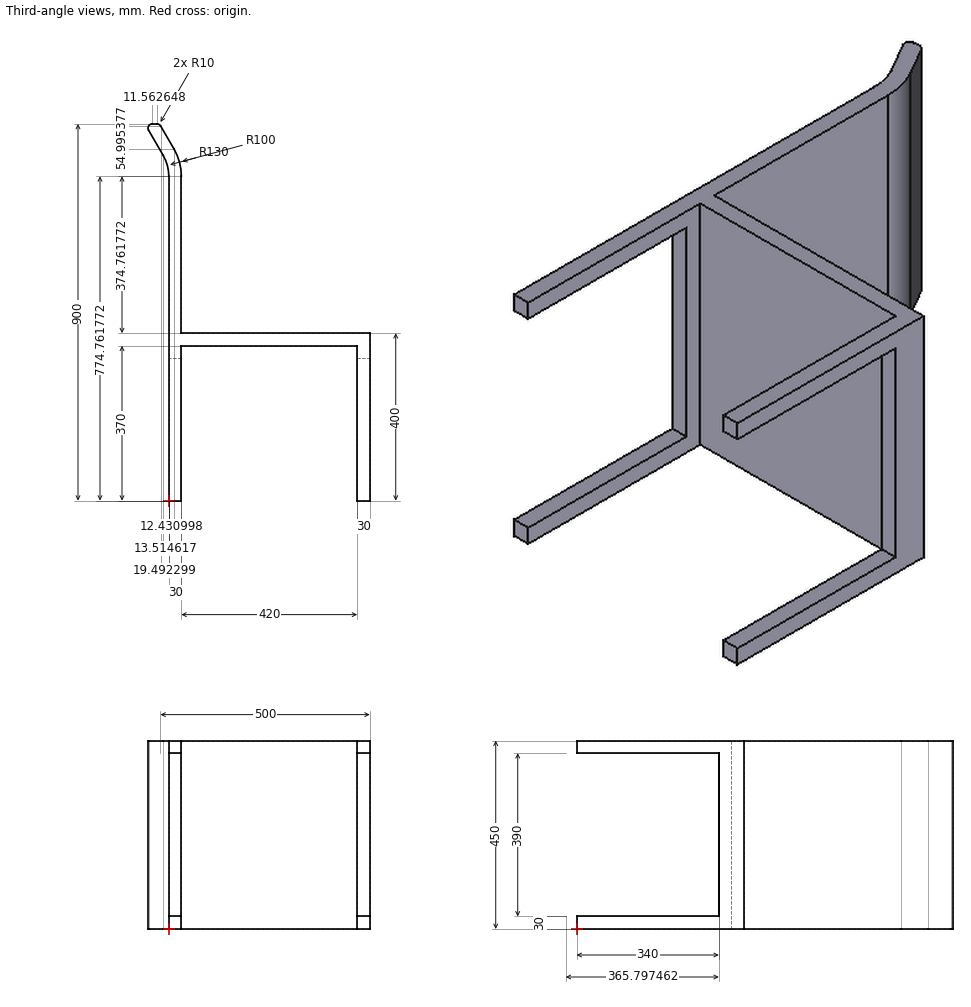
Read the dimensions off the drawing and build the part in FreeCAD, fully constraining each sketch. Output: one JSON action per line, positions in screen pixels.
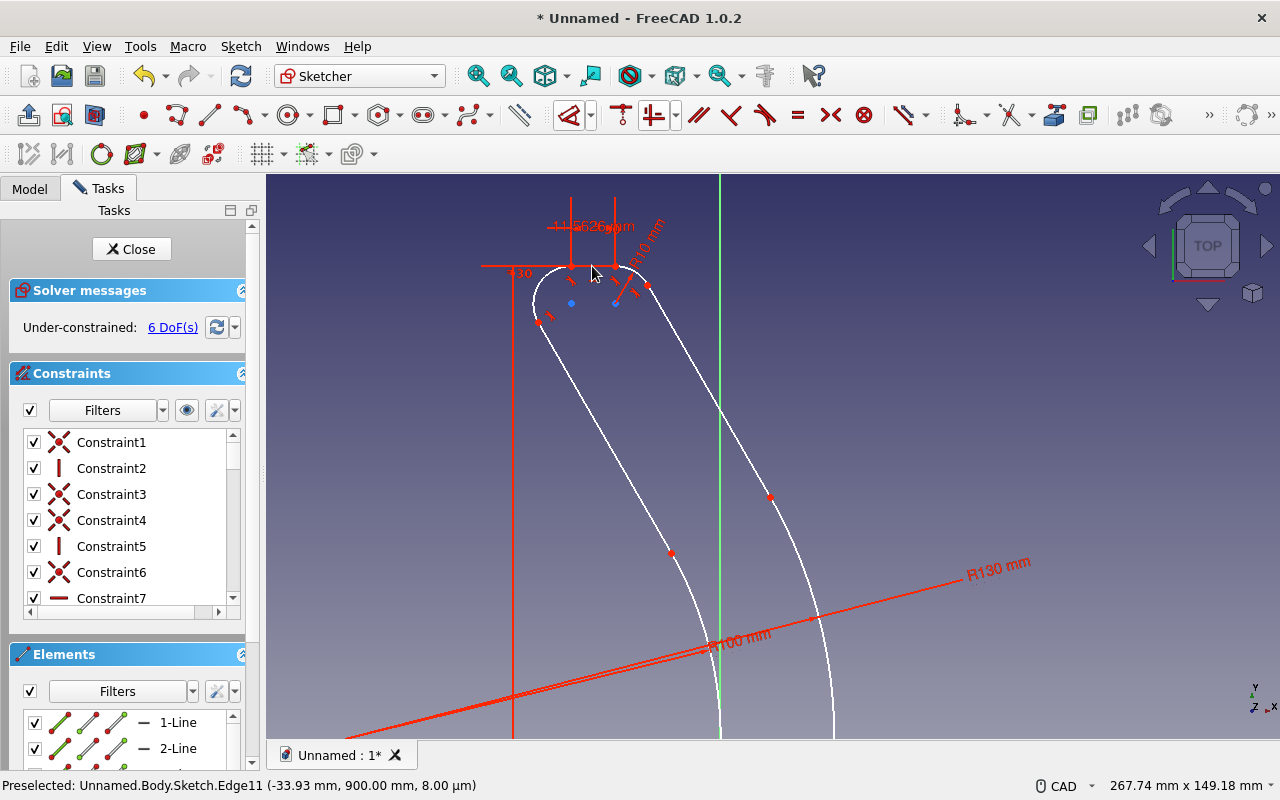
{"action": "scroll", "coordinate": [601, 268], "scroll_direction": "down", "scroll_amount": 11}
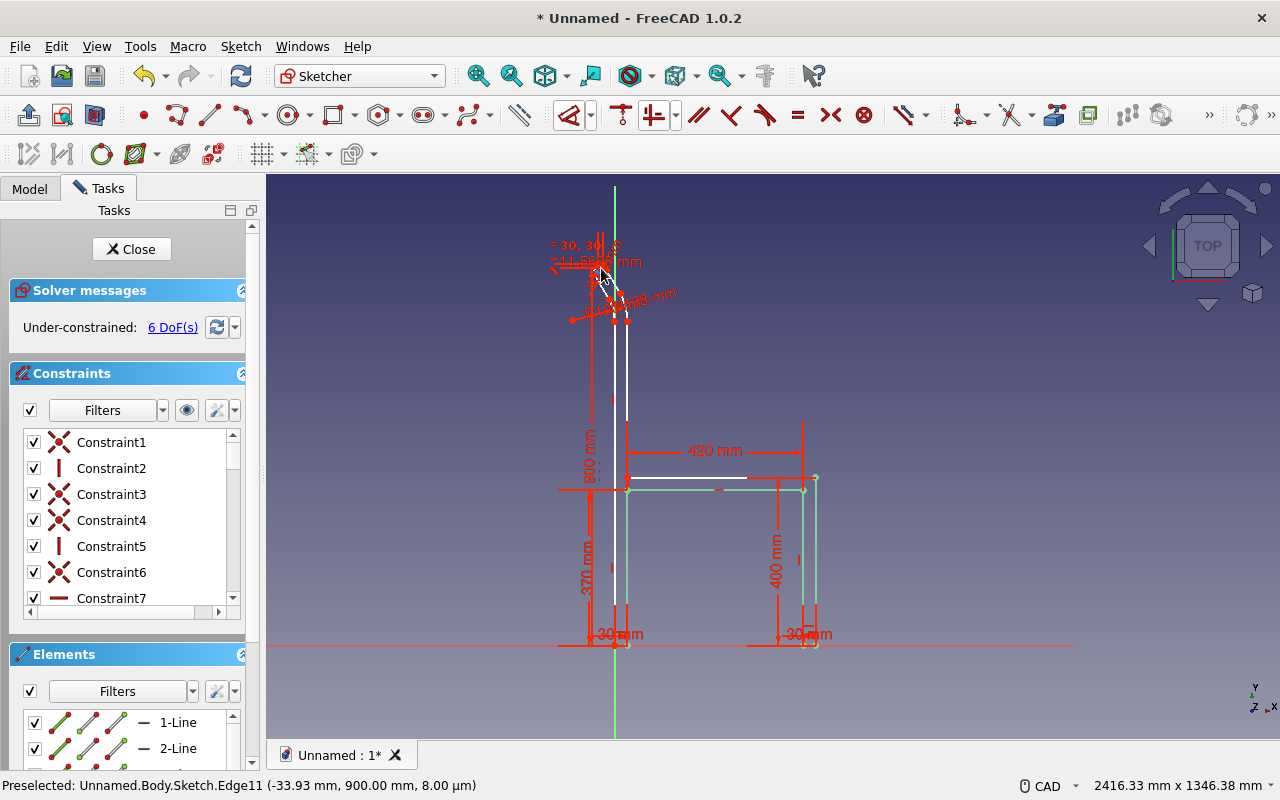
{"action": "left_click", "coordinate": [615, 419]}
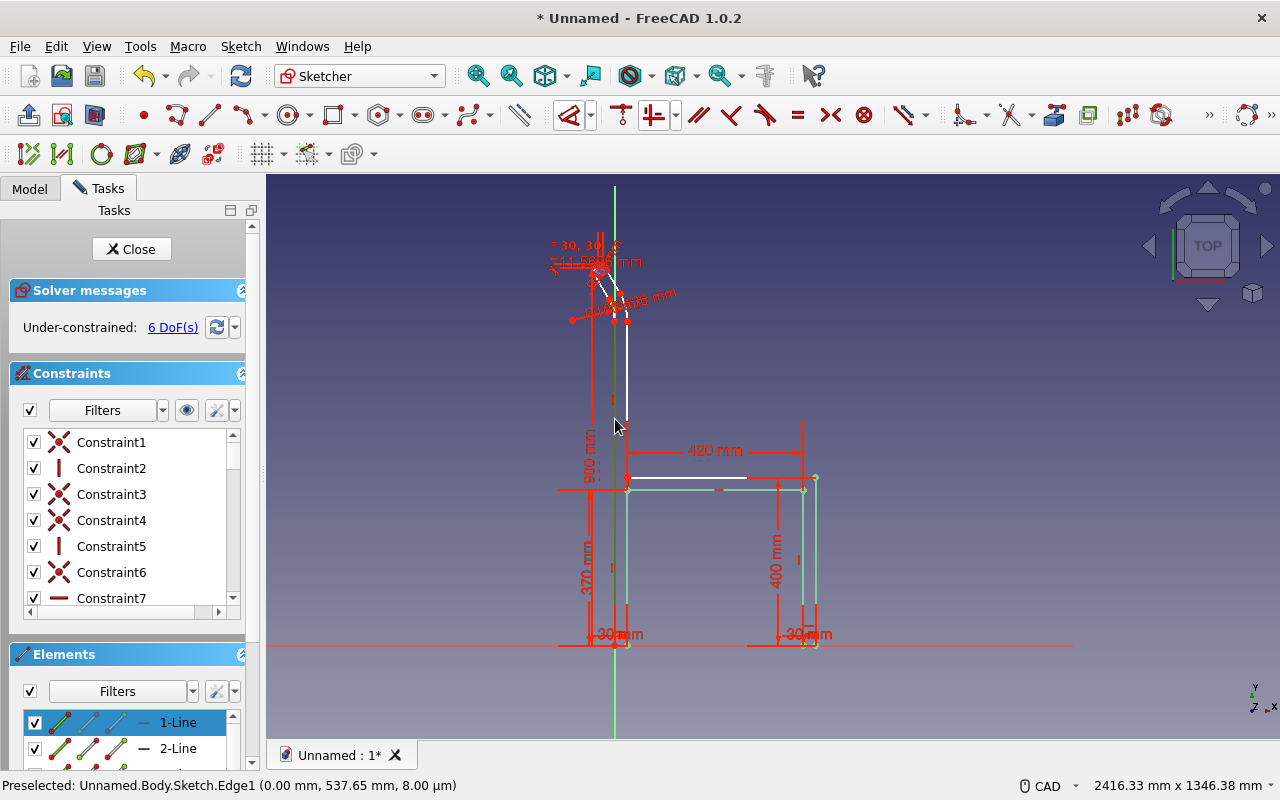
{"action": "key", "text": "i"}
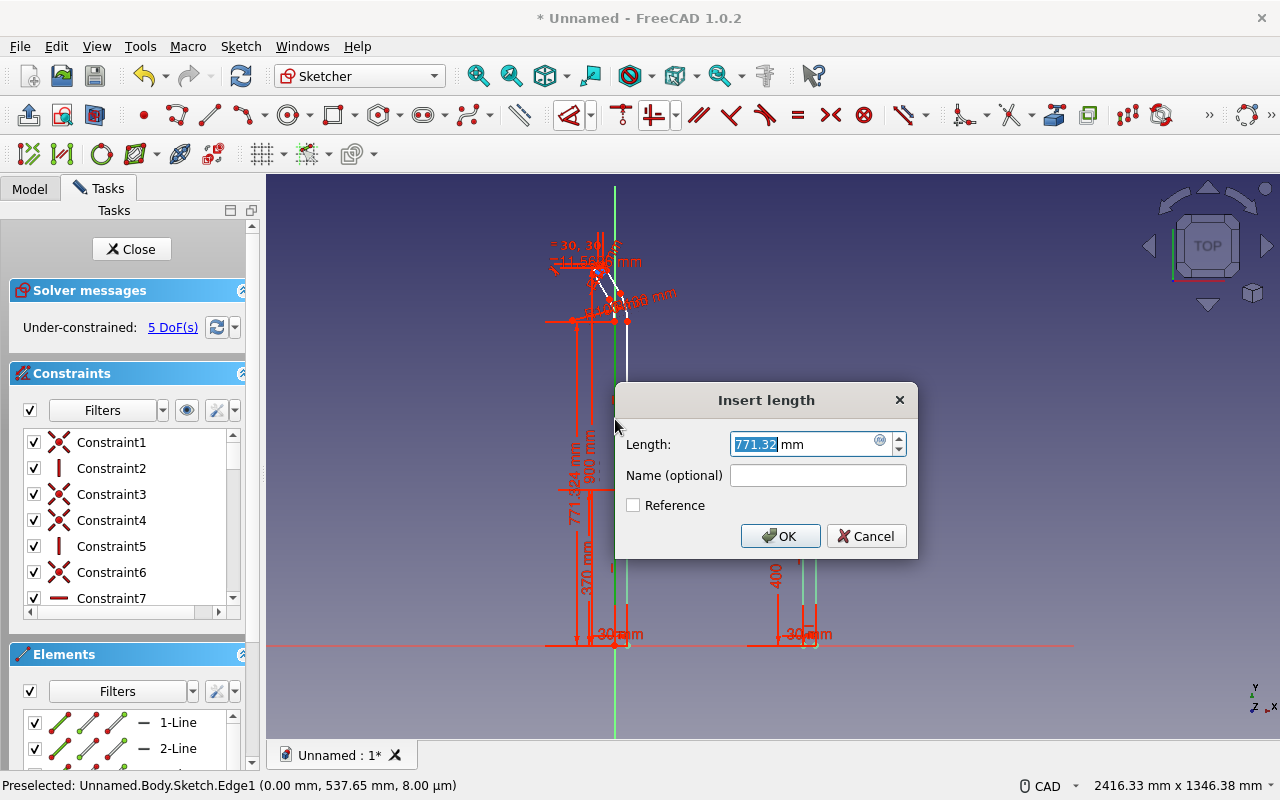
{"action": "type", "text": "774.761772"}
{"action": "key", "text": "Return"}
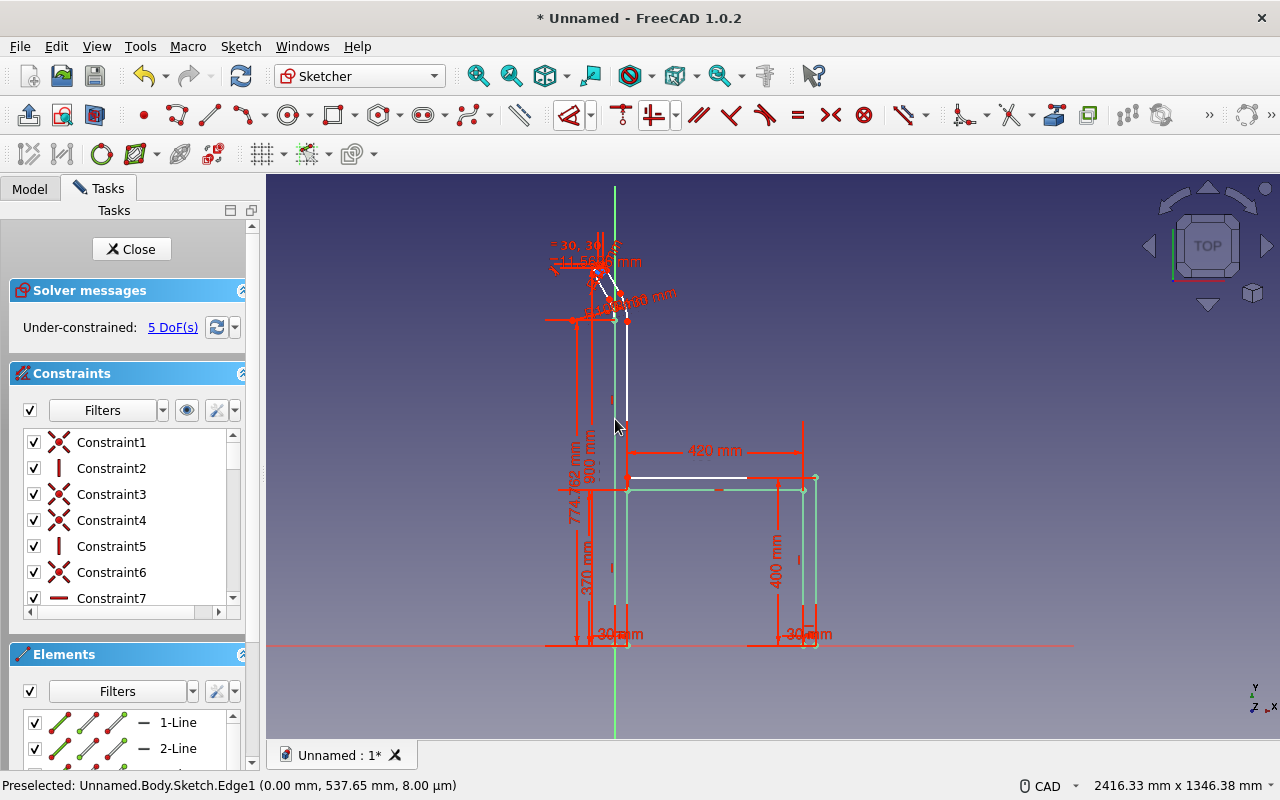
{"action": "left_click", "coordinate": [627, 431]}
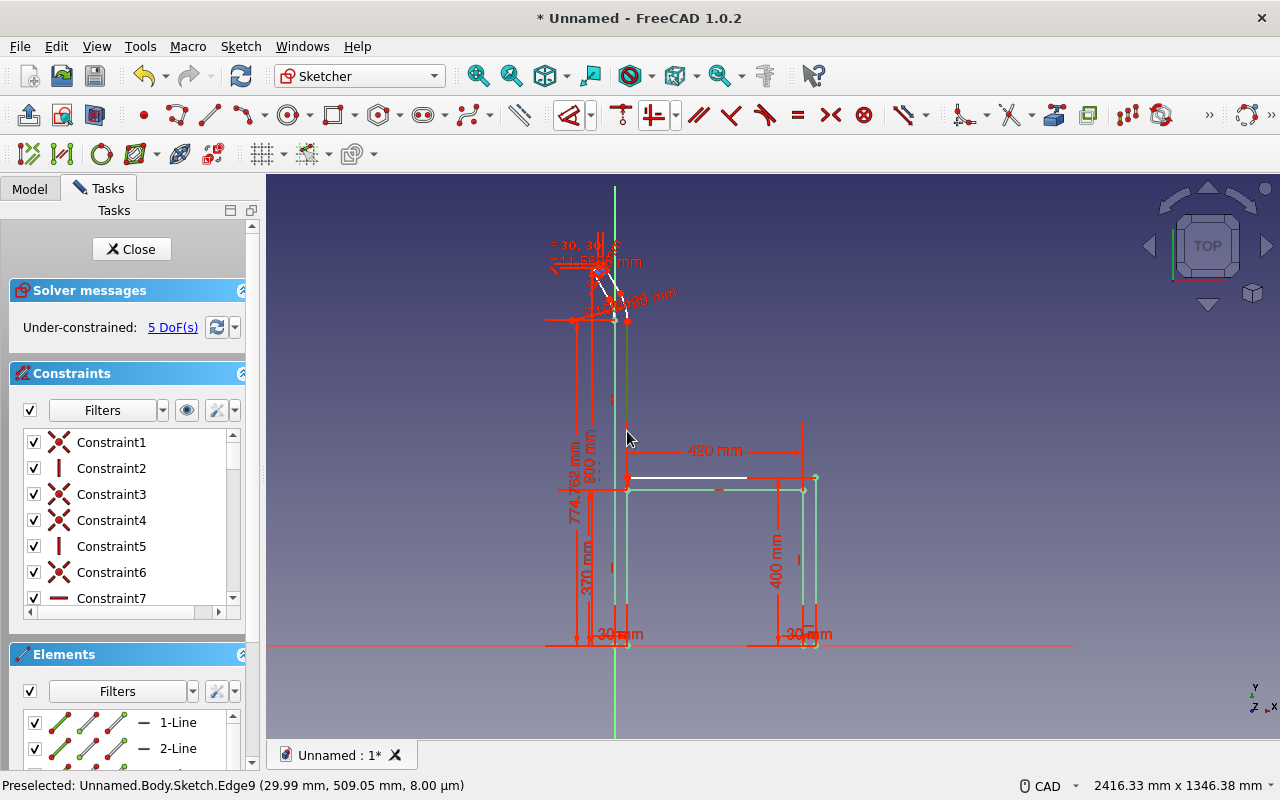
{"action": "key", "text": "i"}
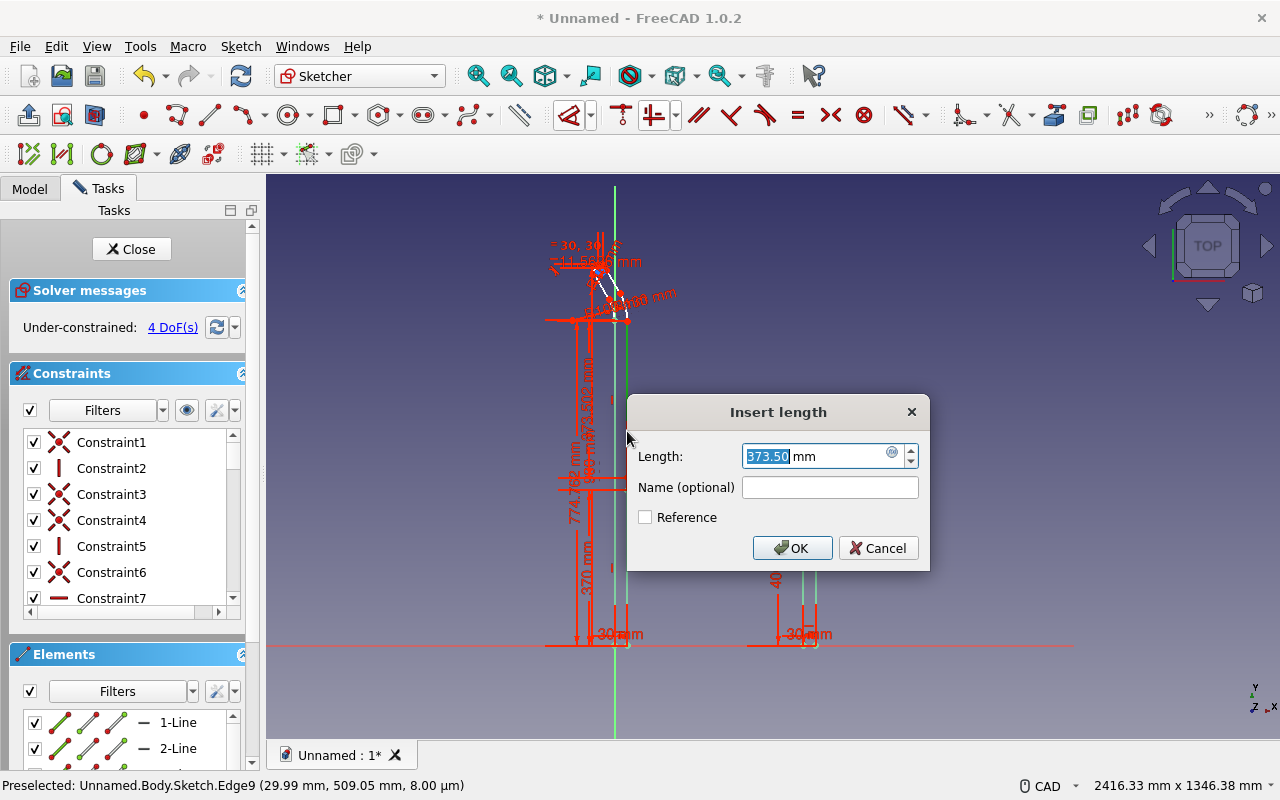
{"action": "type", "text": "374.761772"}
{"action": "key", "text": "Return"}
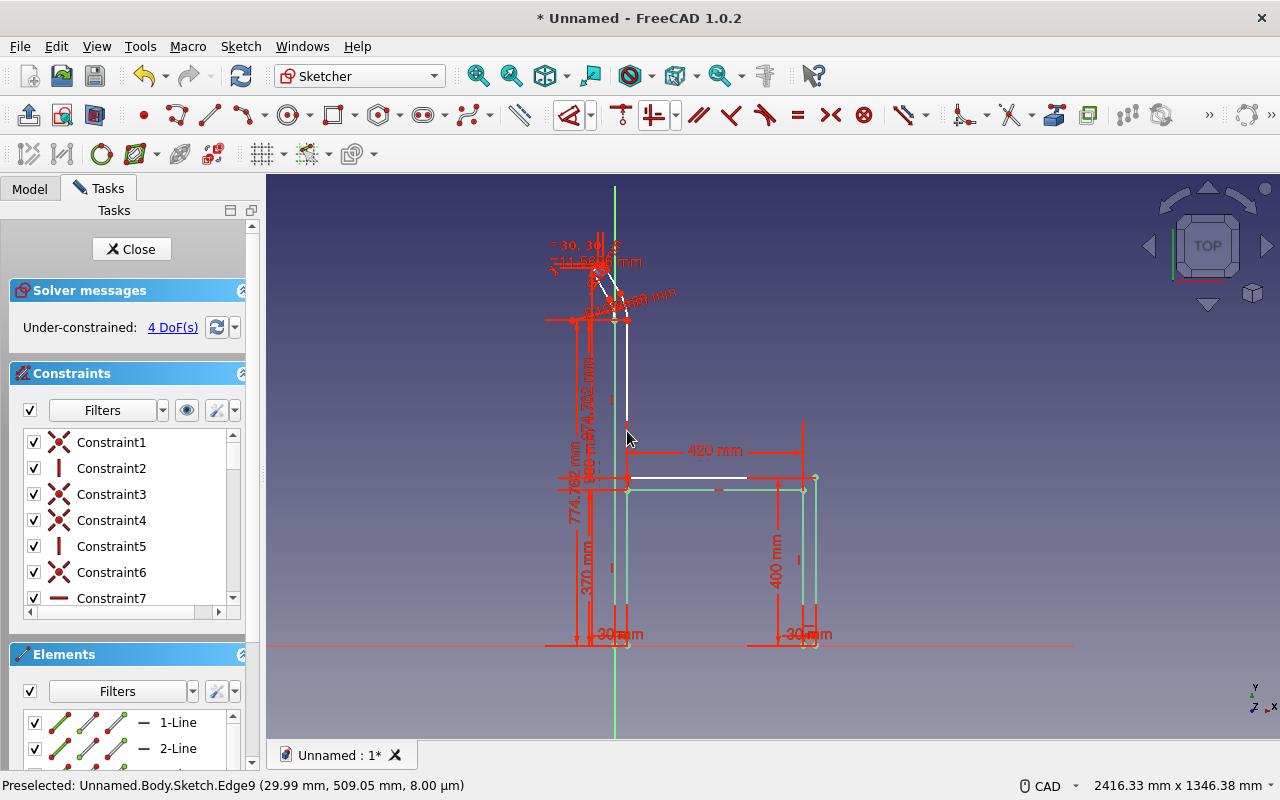
{"action": "scroll", "coordinate": [620, 294], "scroll_direction": "up", "scroll_amount": 11}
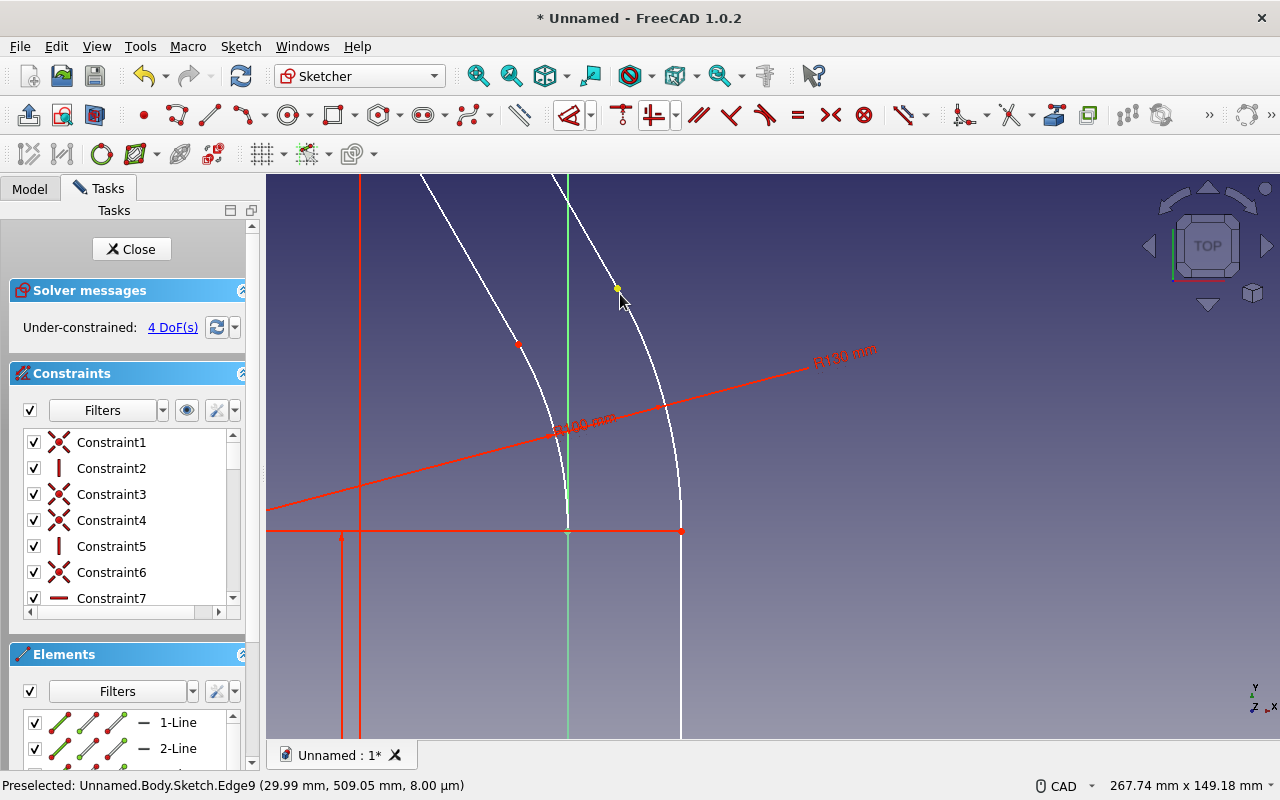
{"action": "left_click", "coordinate": [618, 288]}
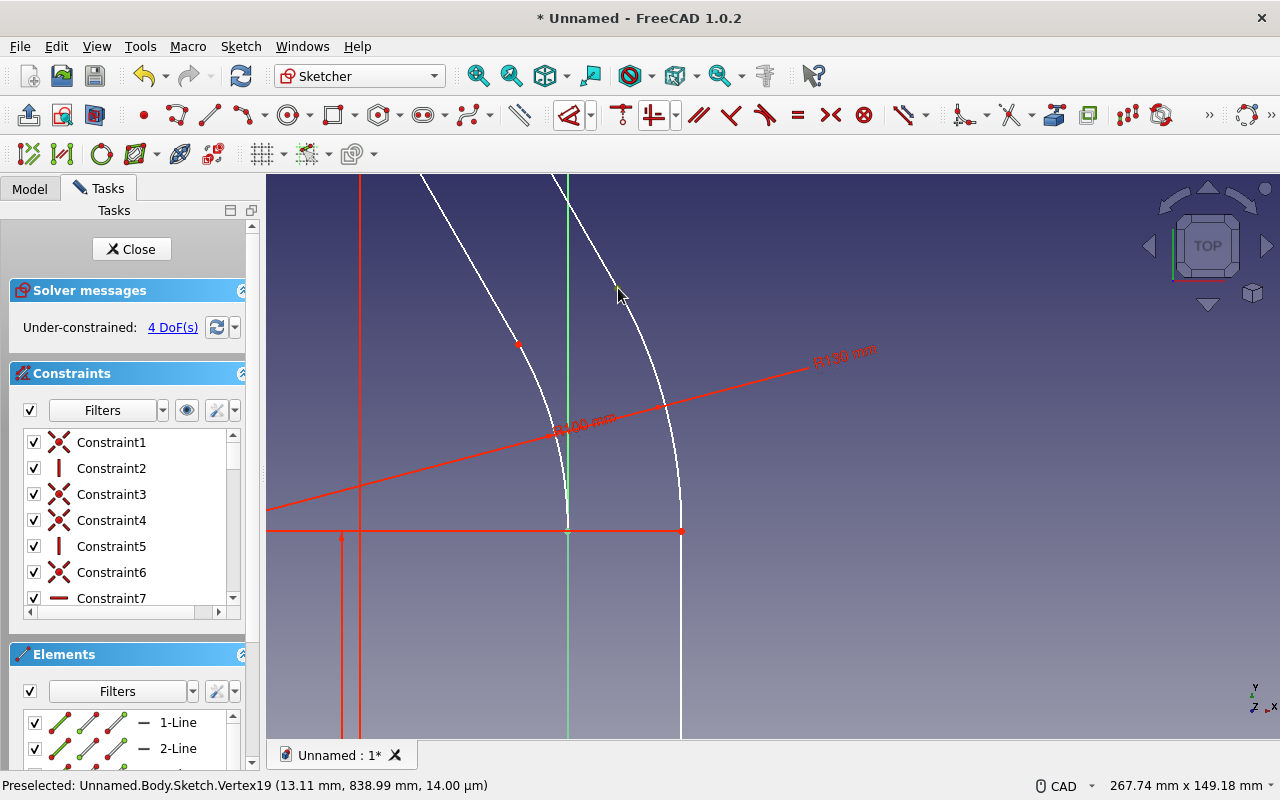
{"action": "left_click", "coordinate": [590, 116]}